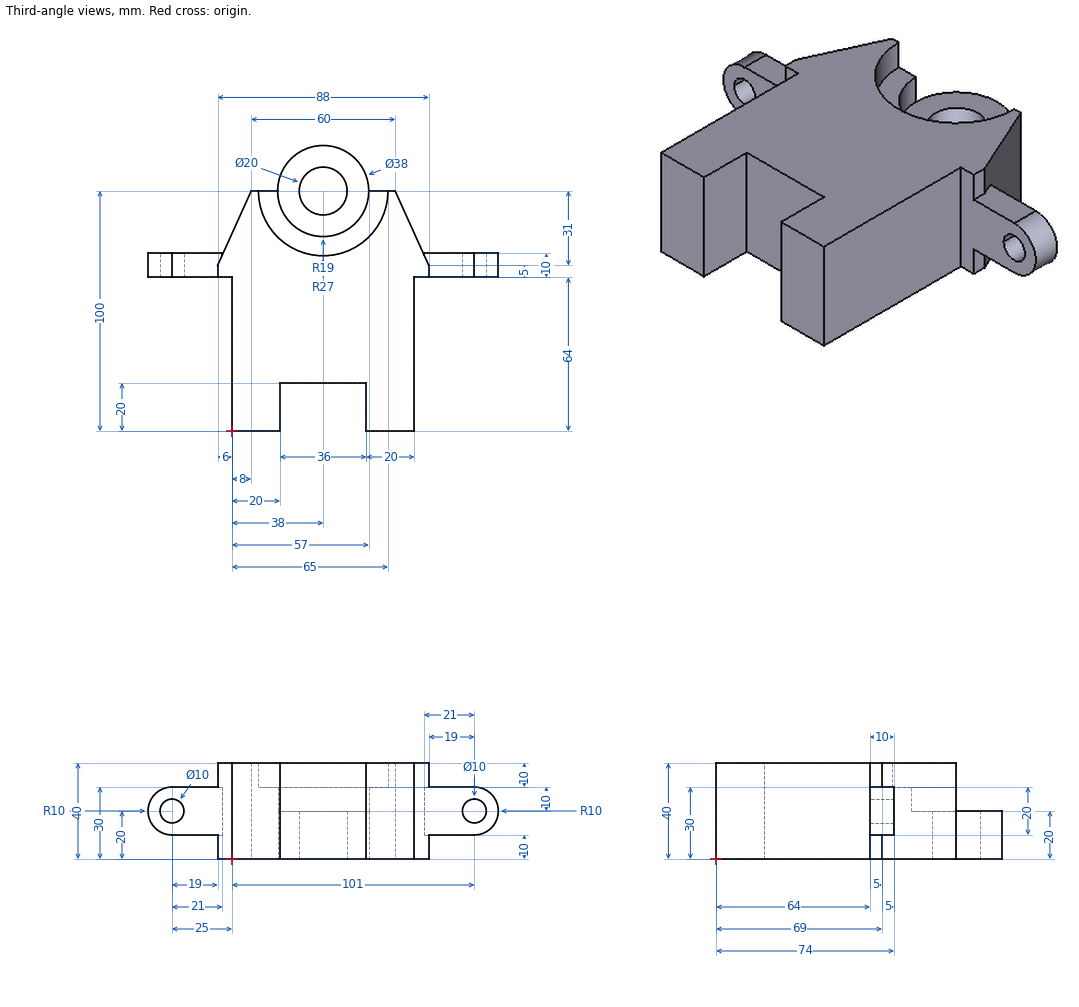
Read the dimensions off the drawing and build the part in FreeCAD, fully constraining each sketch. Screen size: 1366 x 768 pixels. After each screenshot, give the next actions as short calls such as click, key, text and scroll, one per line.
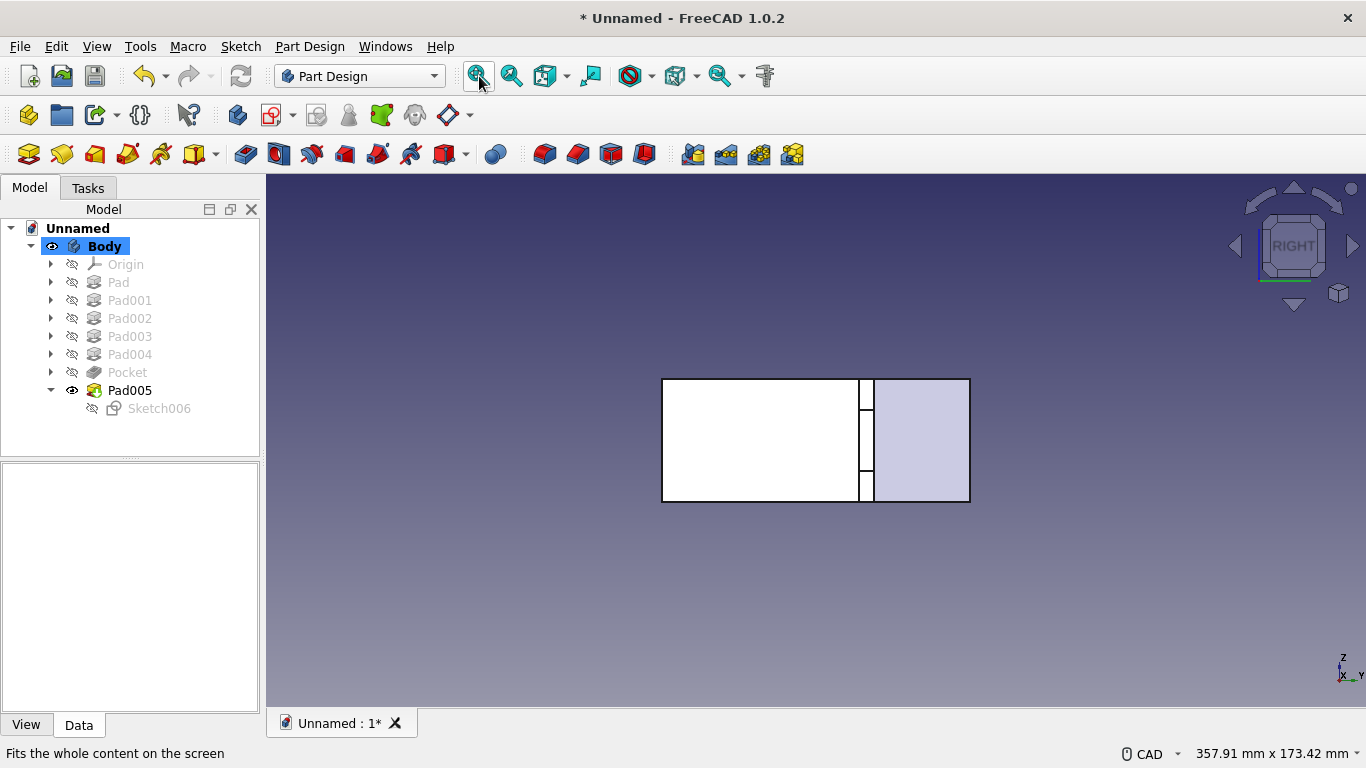
click(479, 76)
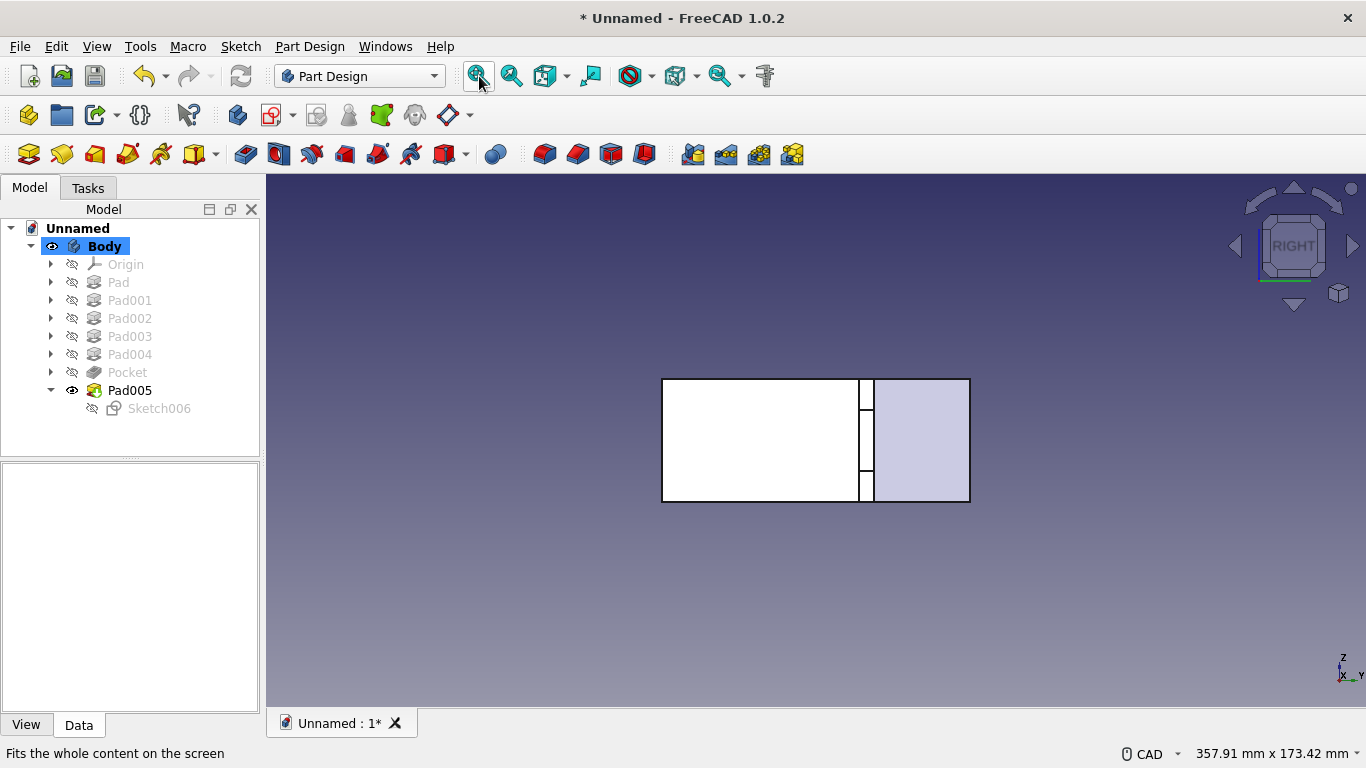
key(2)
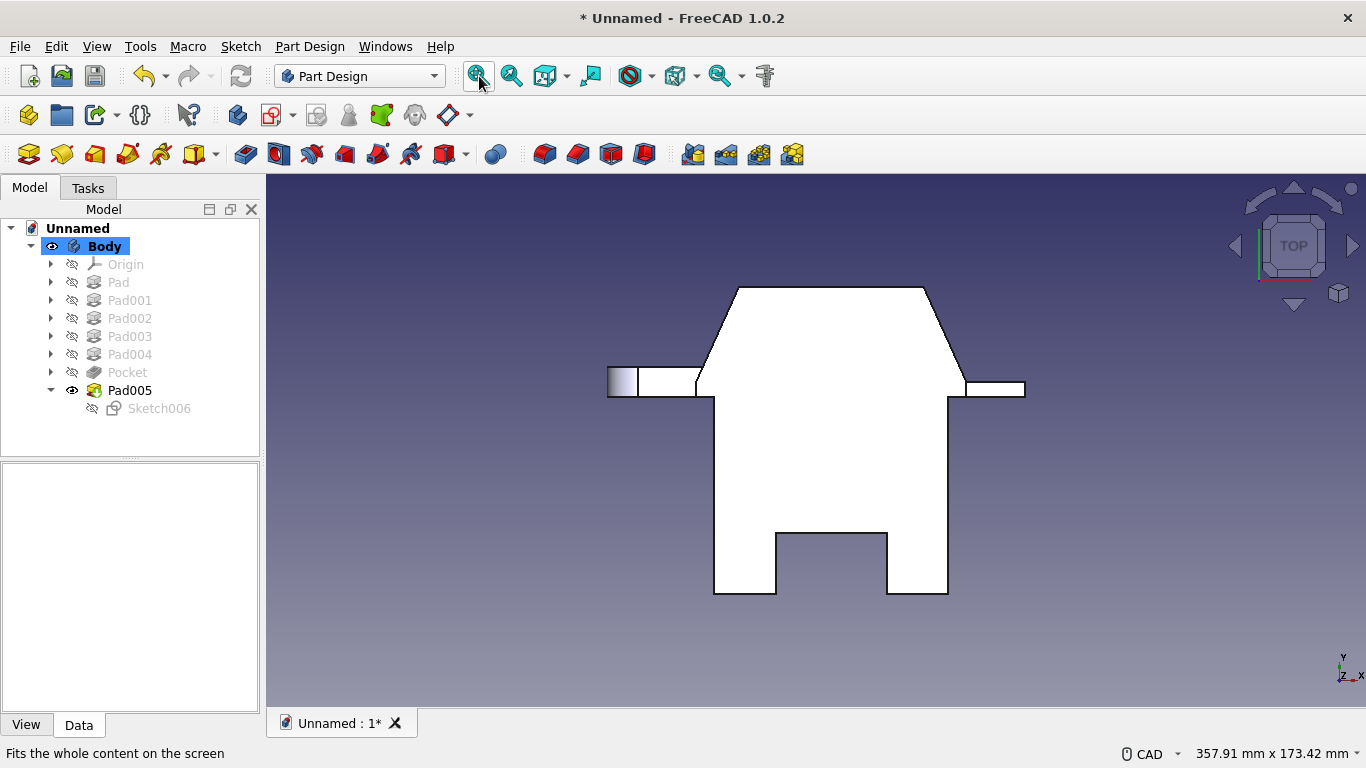
click(51, 264)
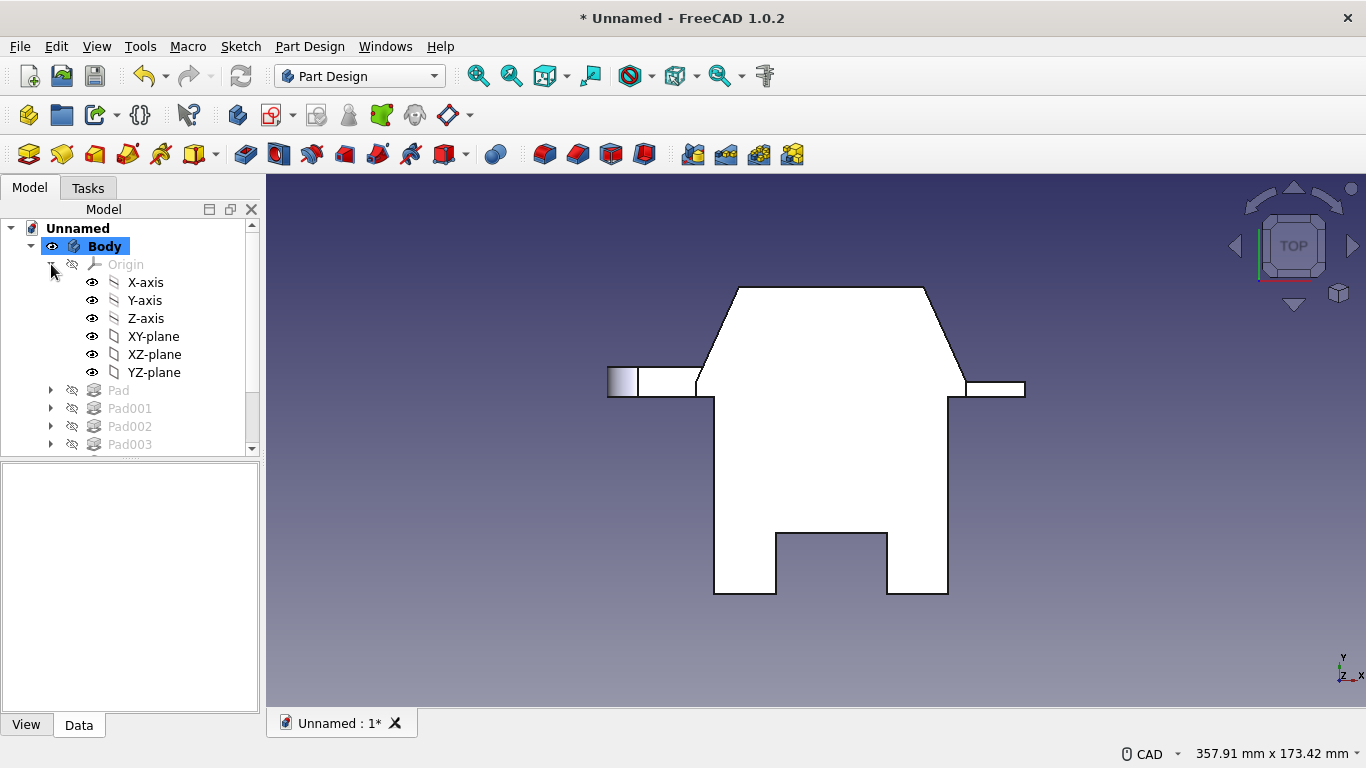
click(137, 372)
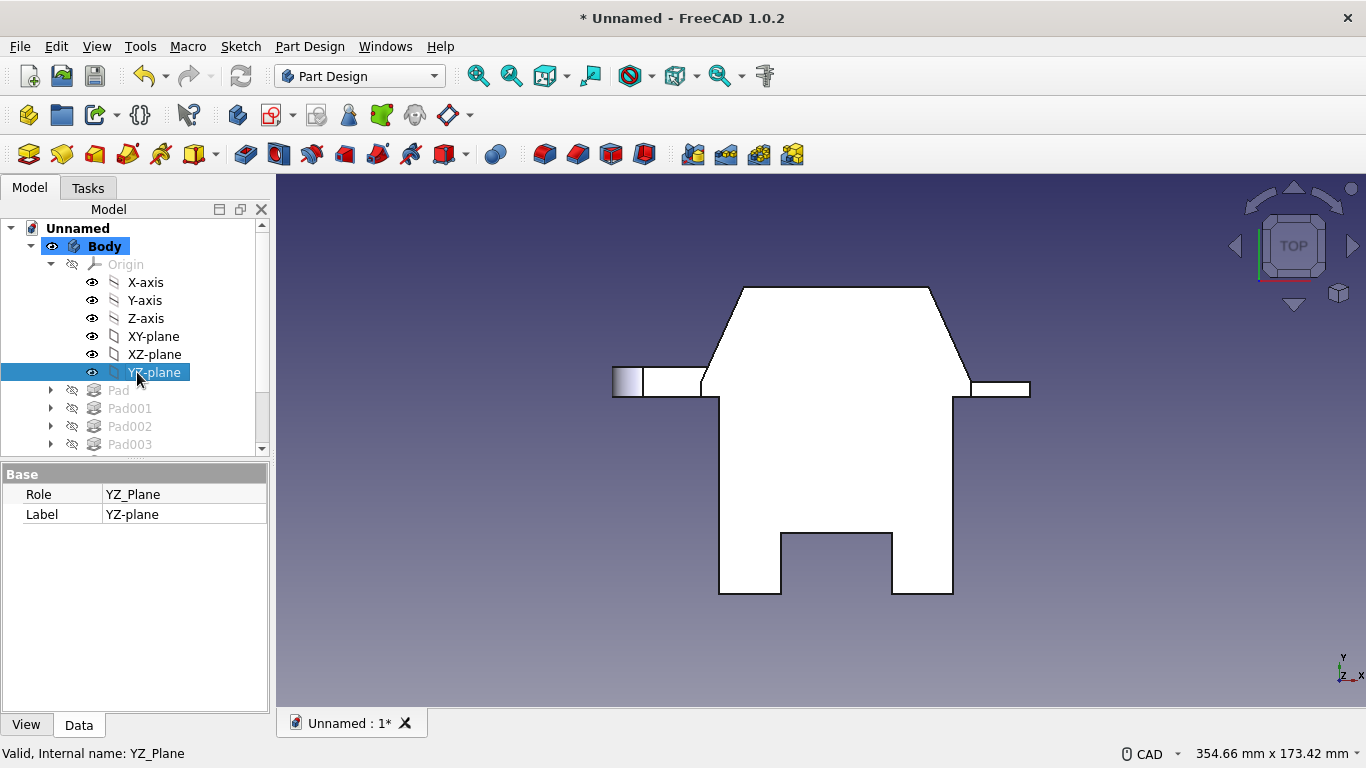
click(448, 116)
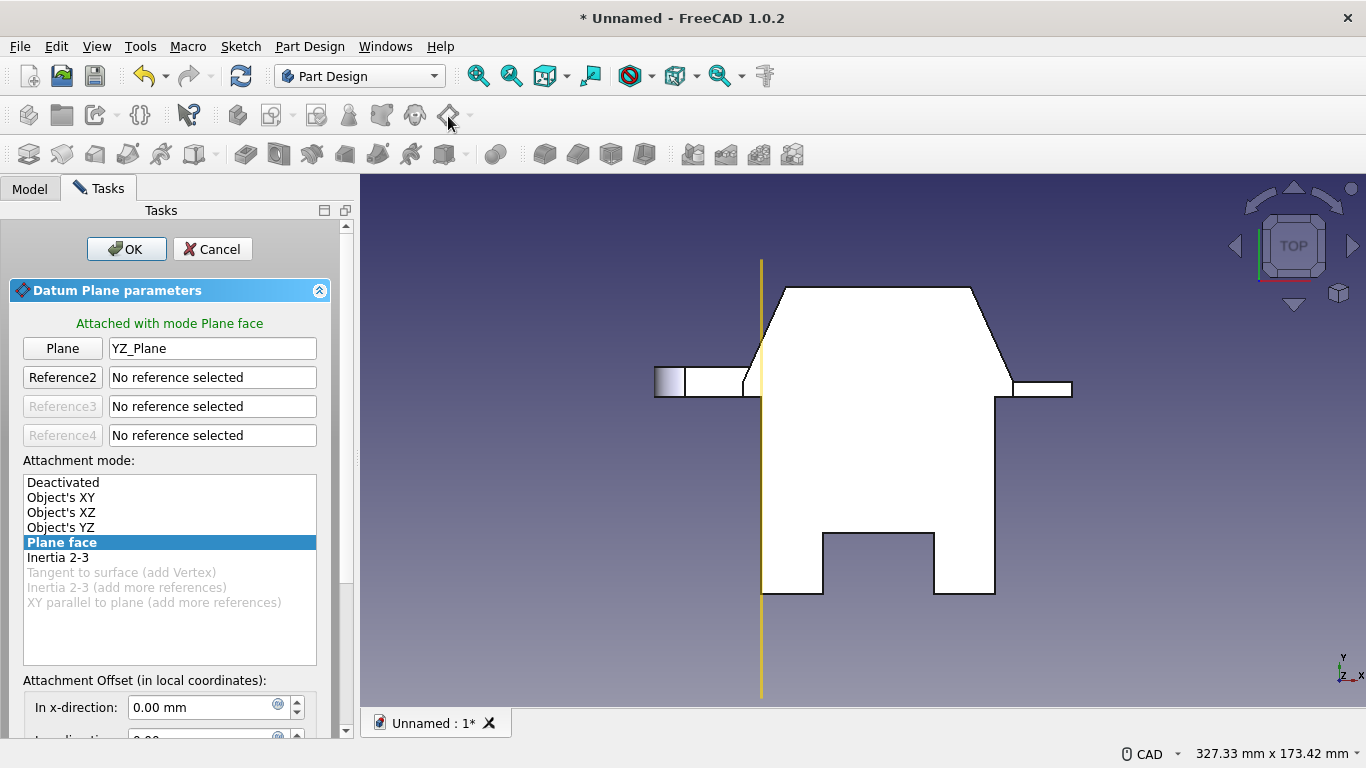
scroll(346, 479, down, 2)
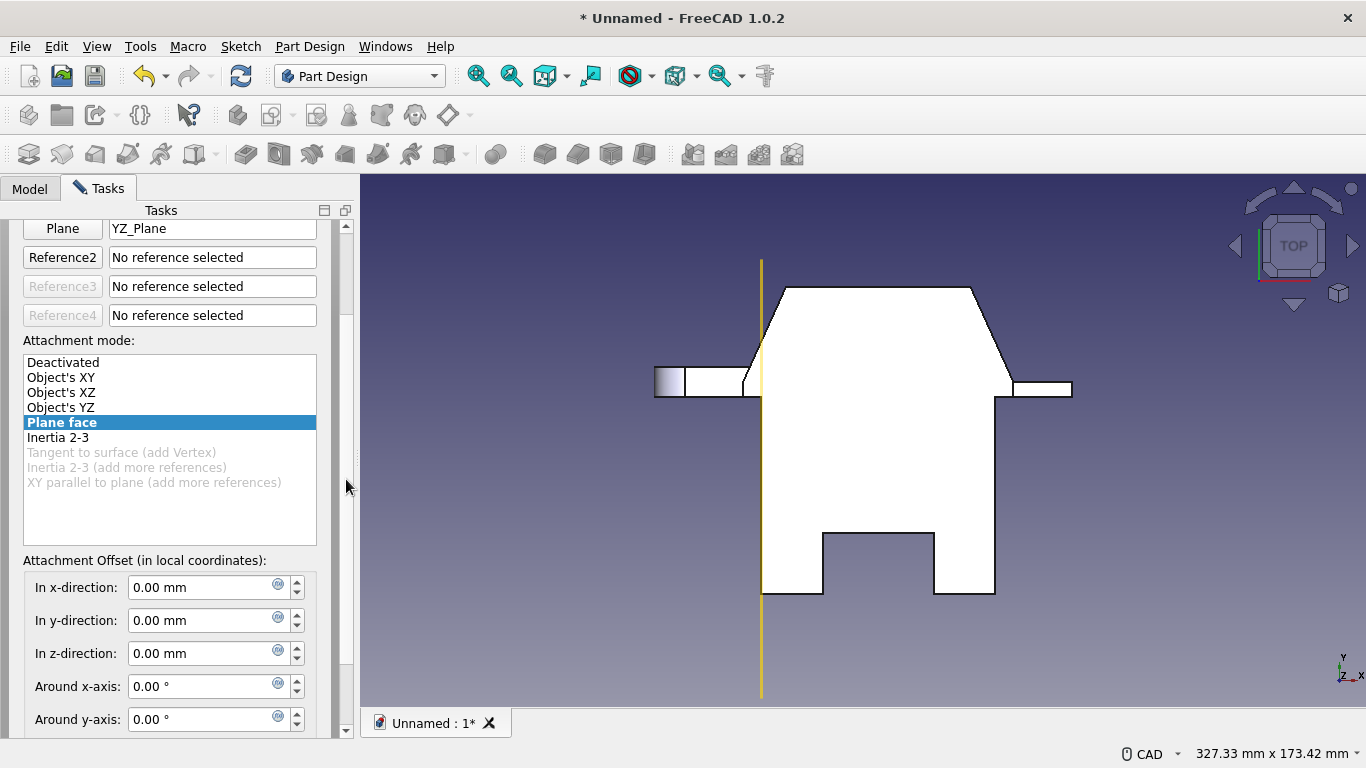
triple_click(210, 654)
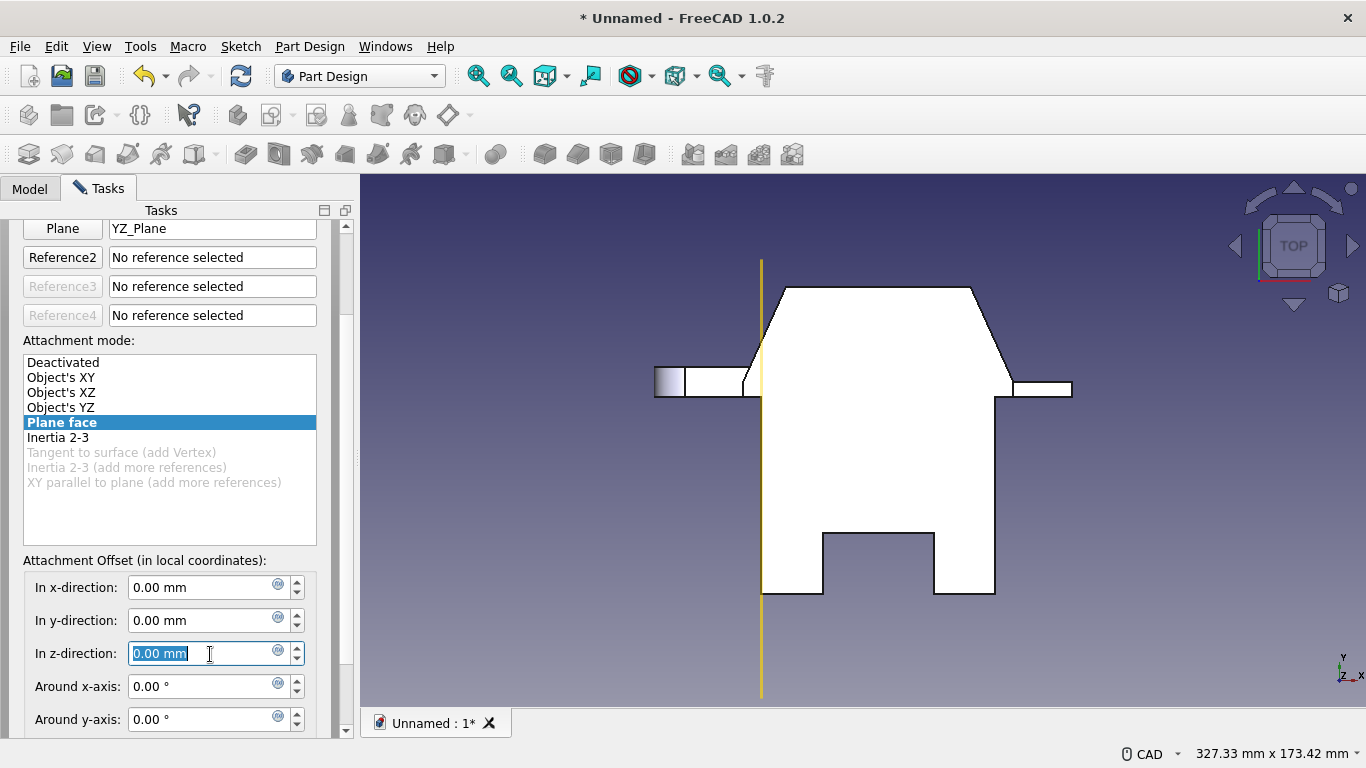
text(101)
key(Tab)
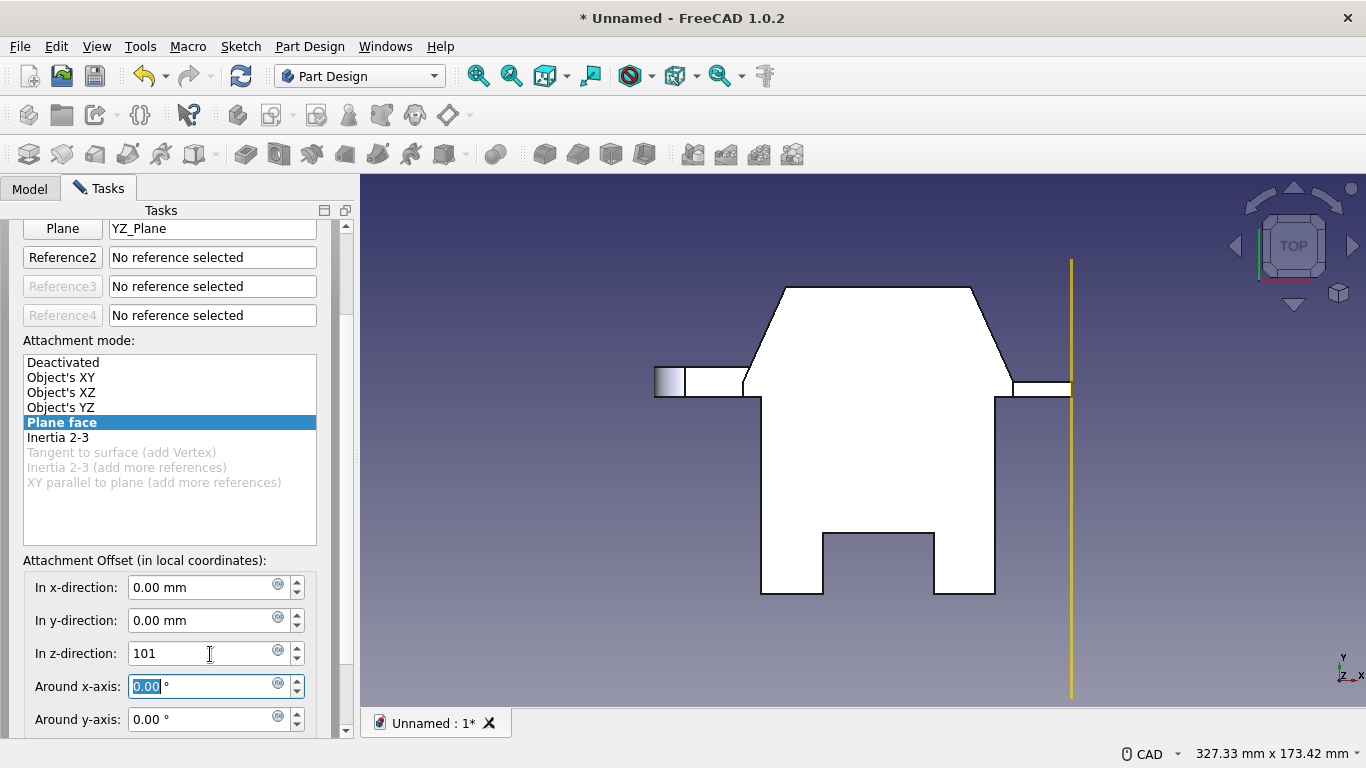
scroll(346, 479, up, 3)